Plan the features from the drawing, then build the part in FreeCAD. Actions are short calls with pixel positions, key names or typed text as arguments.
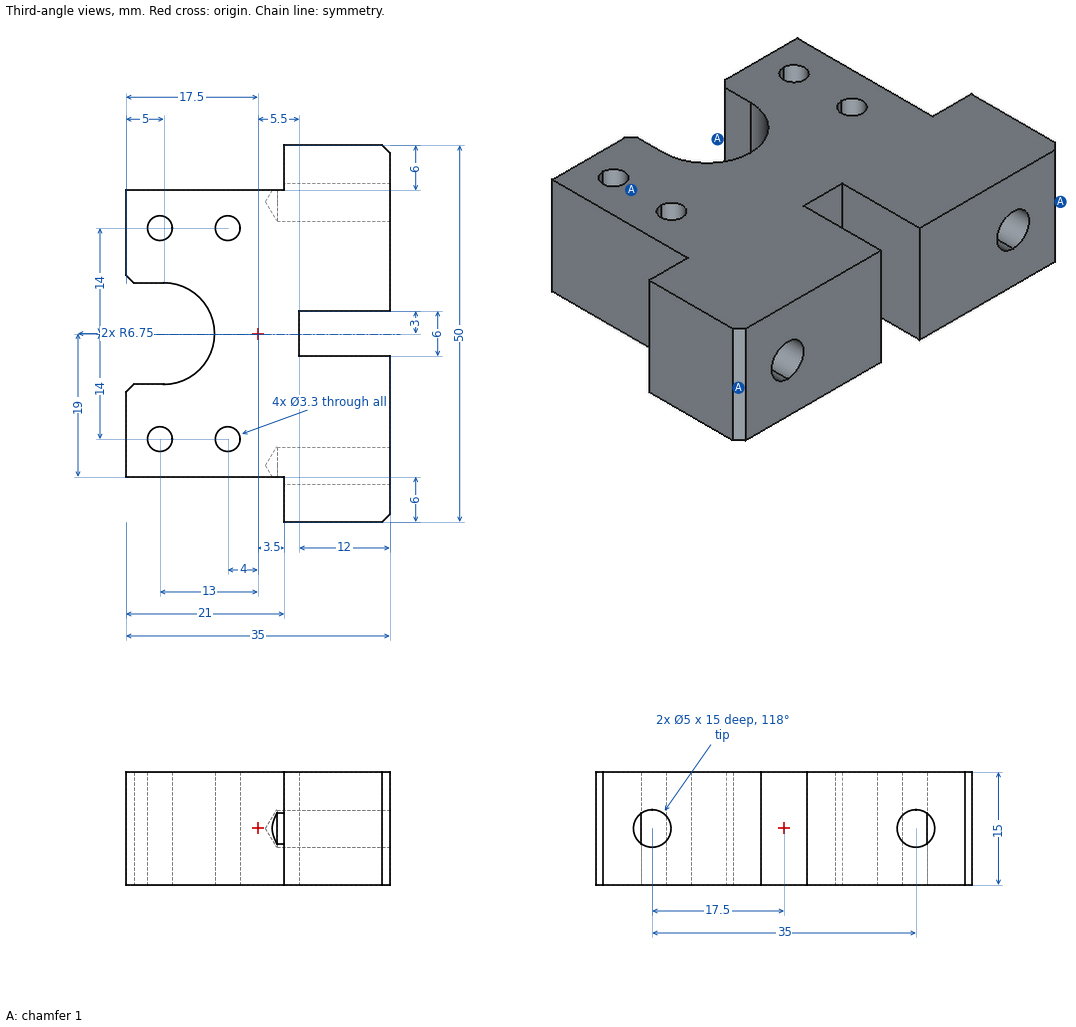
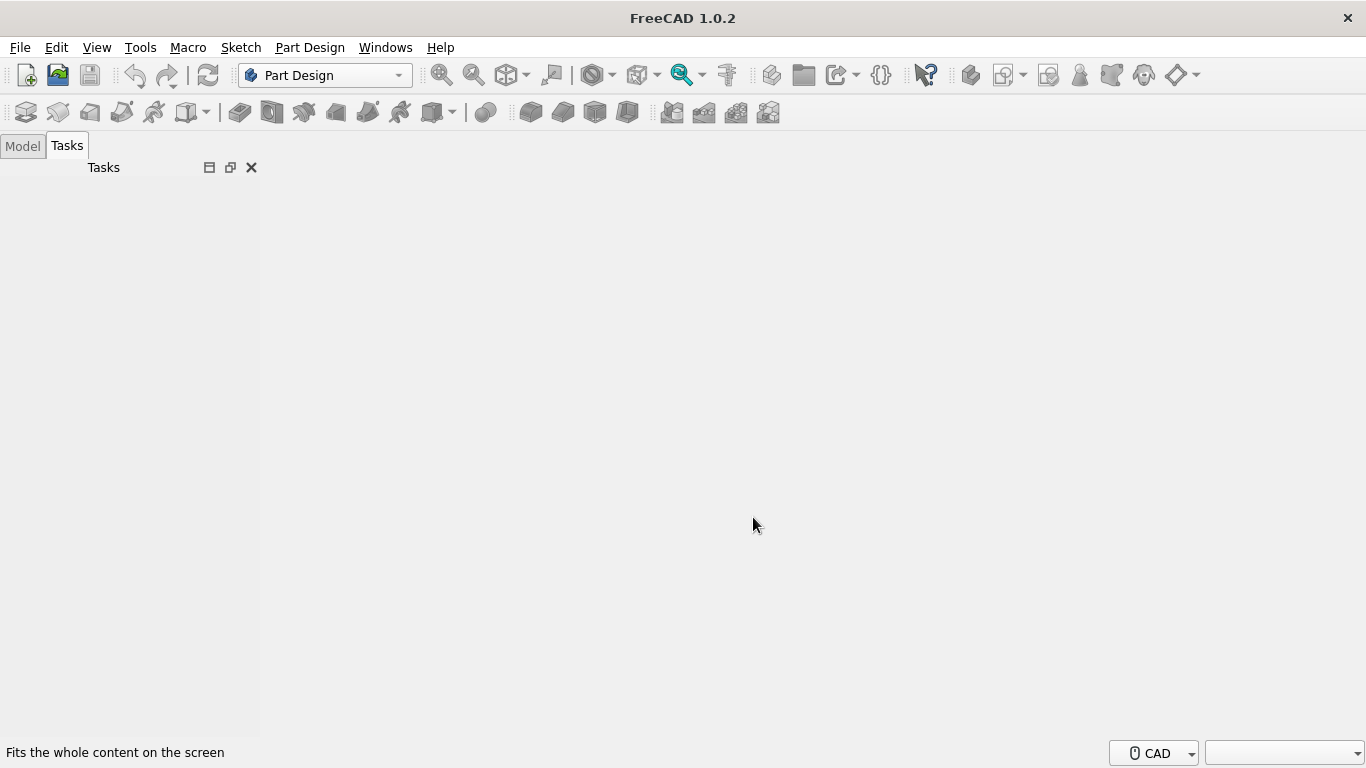
click(26, 76)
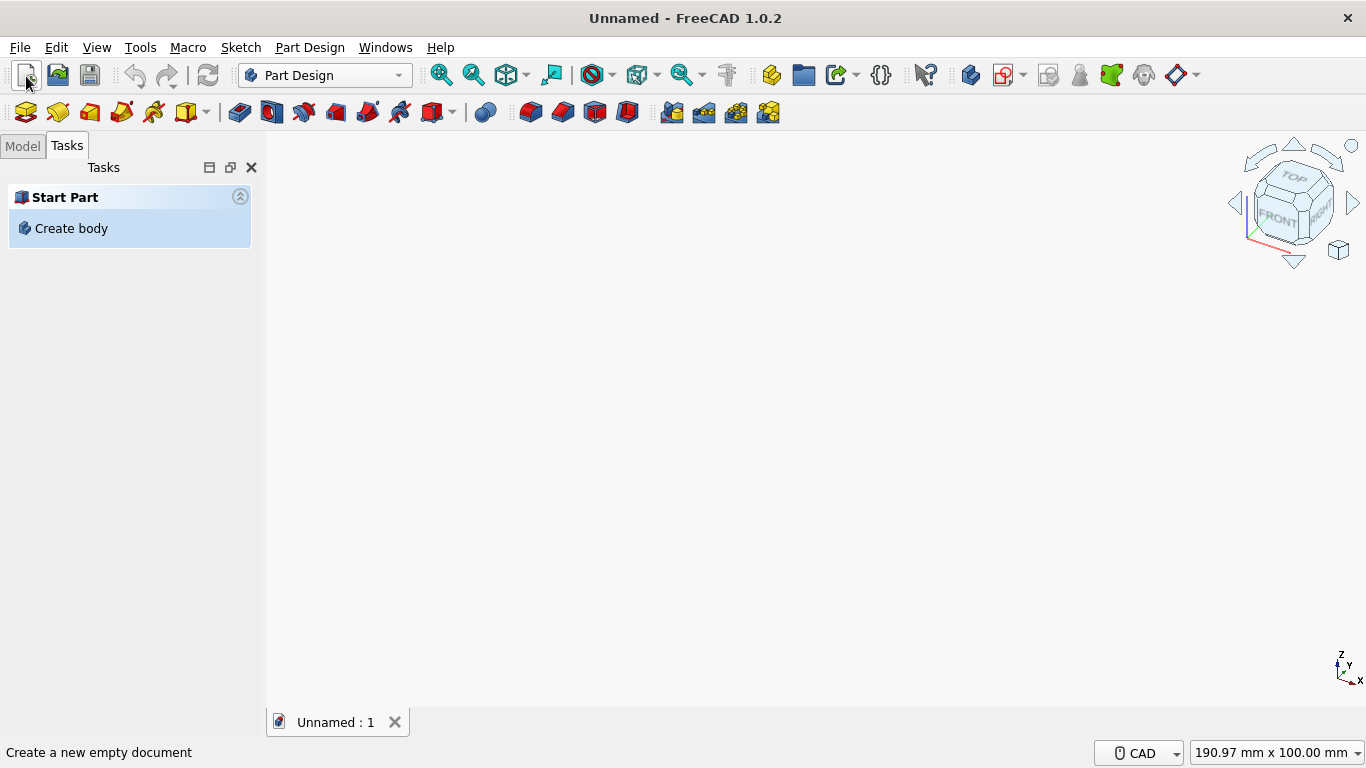
click(1004, 76)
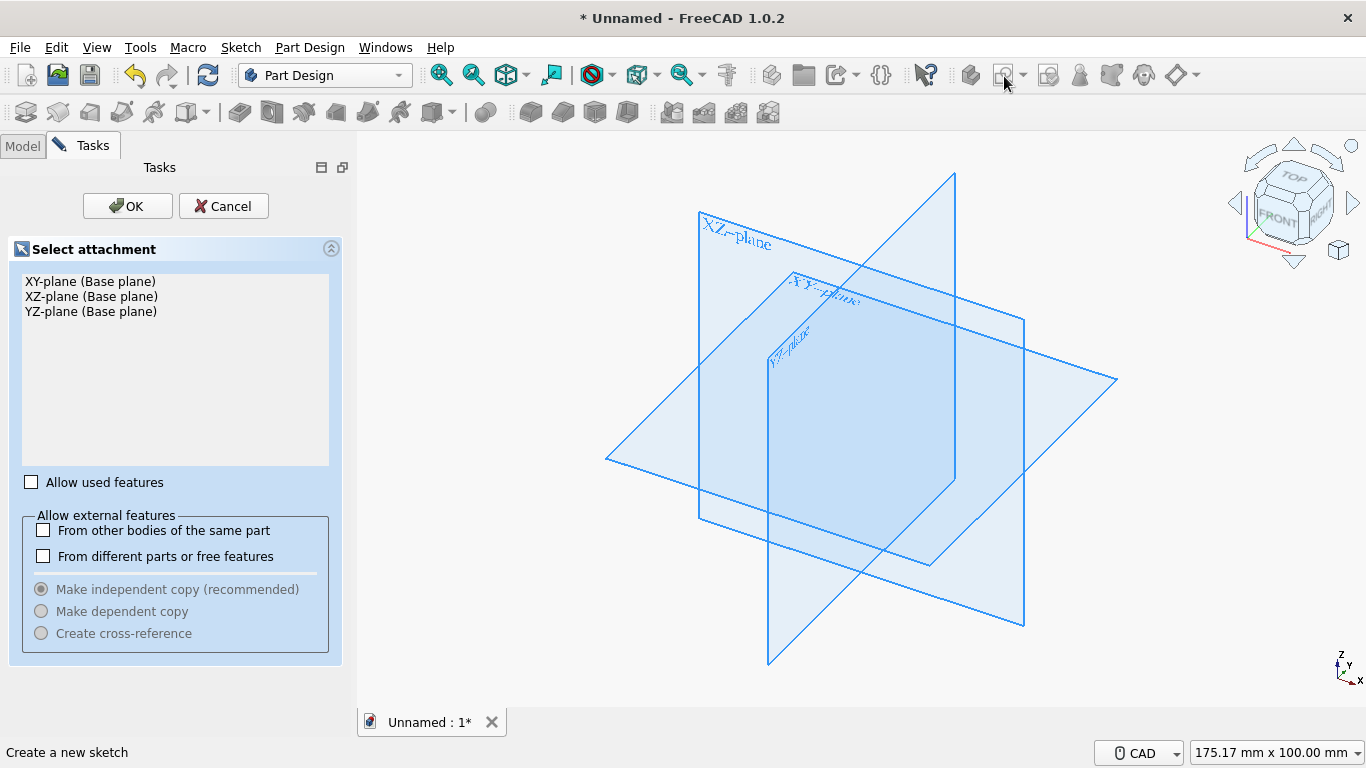
click(82, 282)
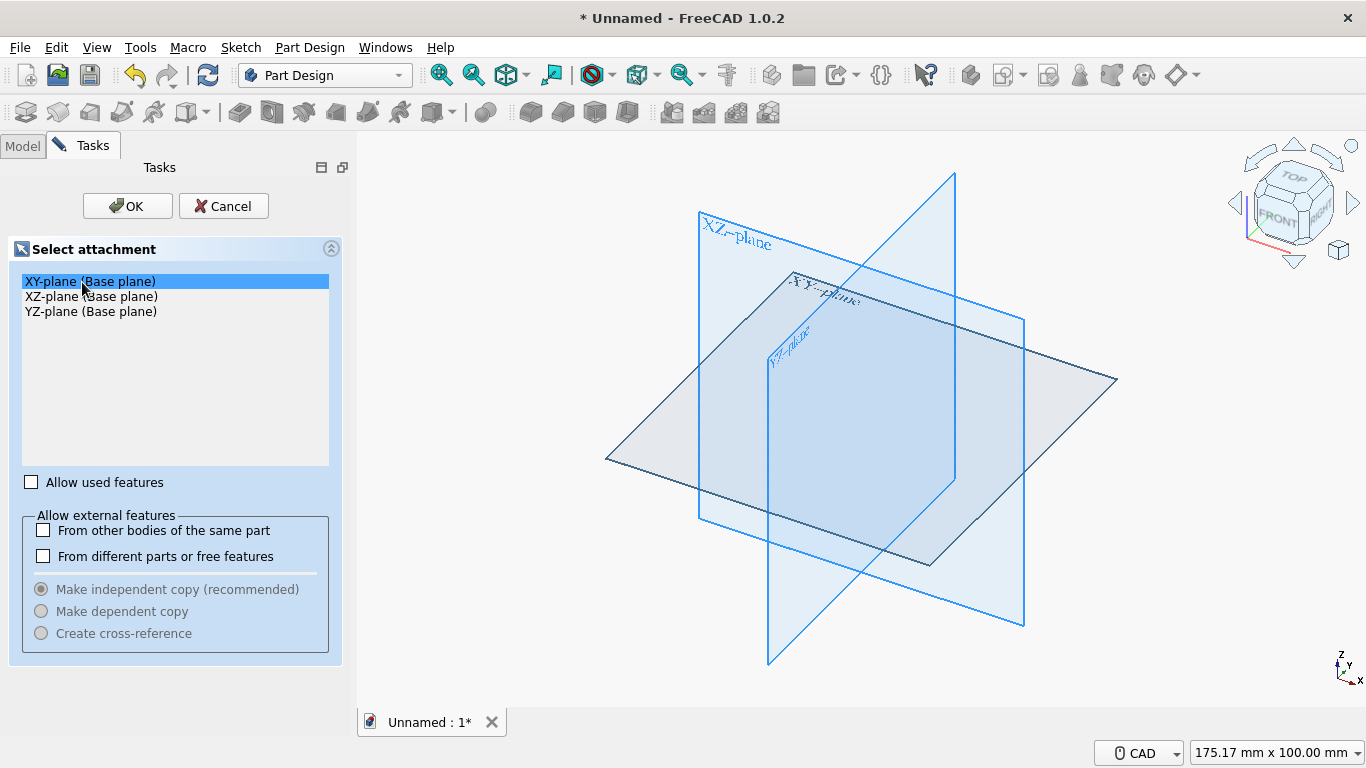
click(128, 206)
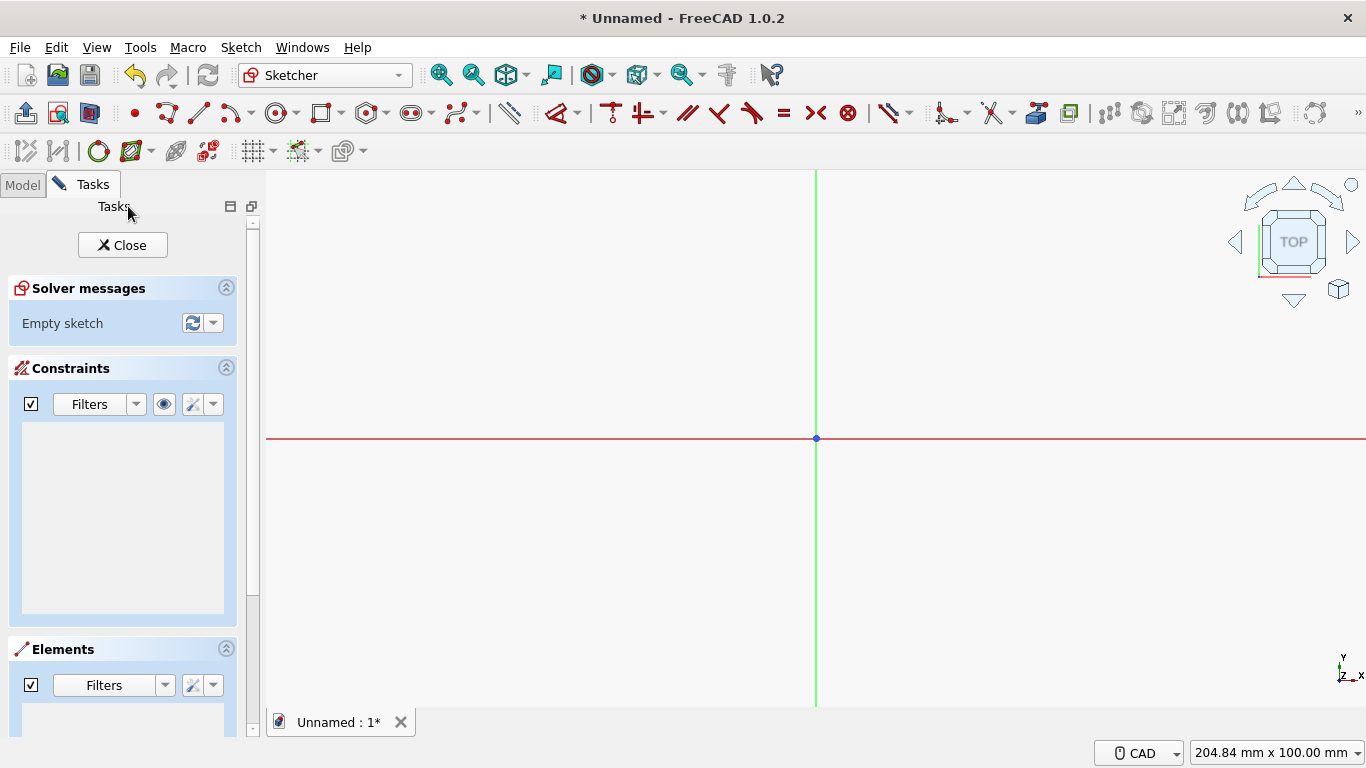
click(344, 114)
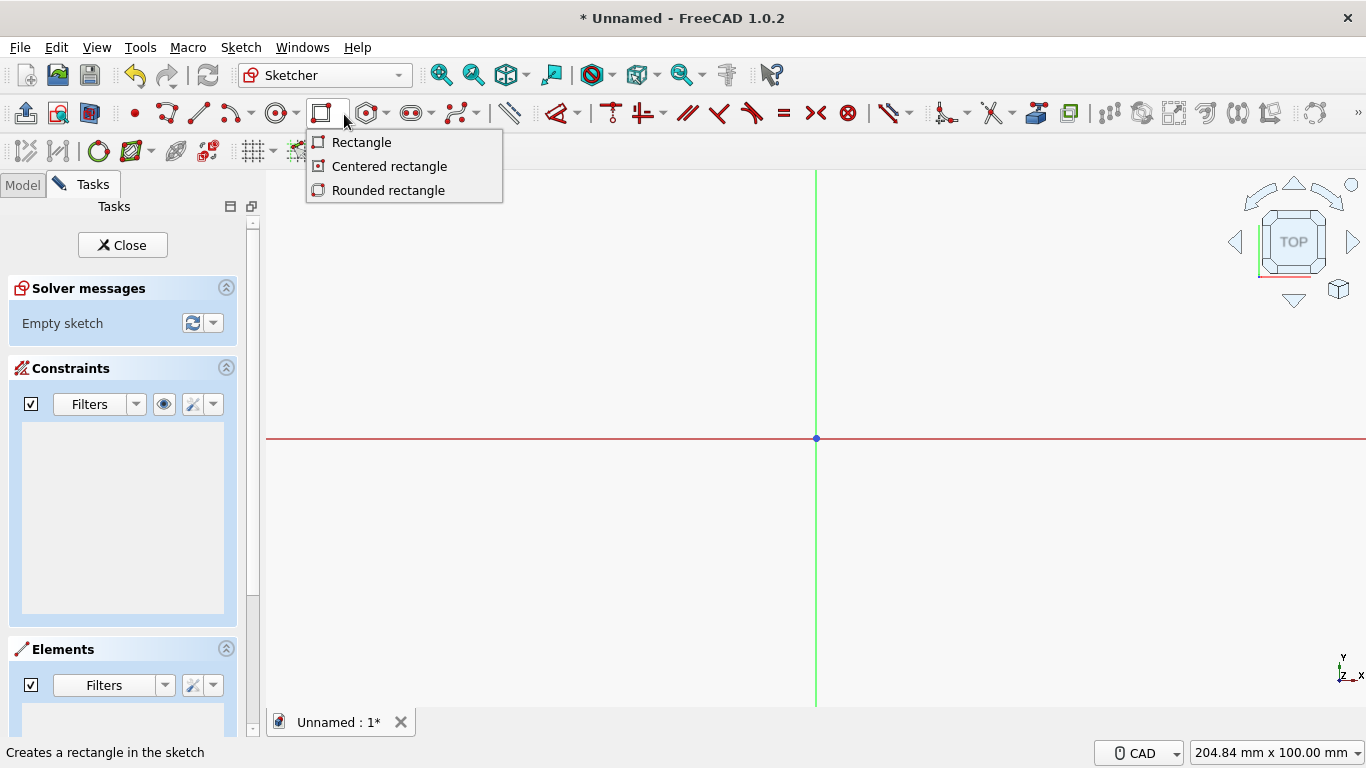
click(404, 166)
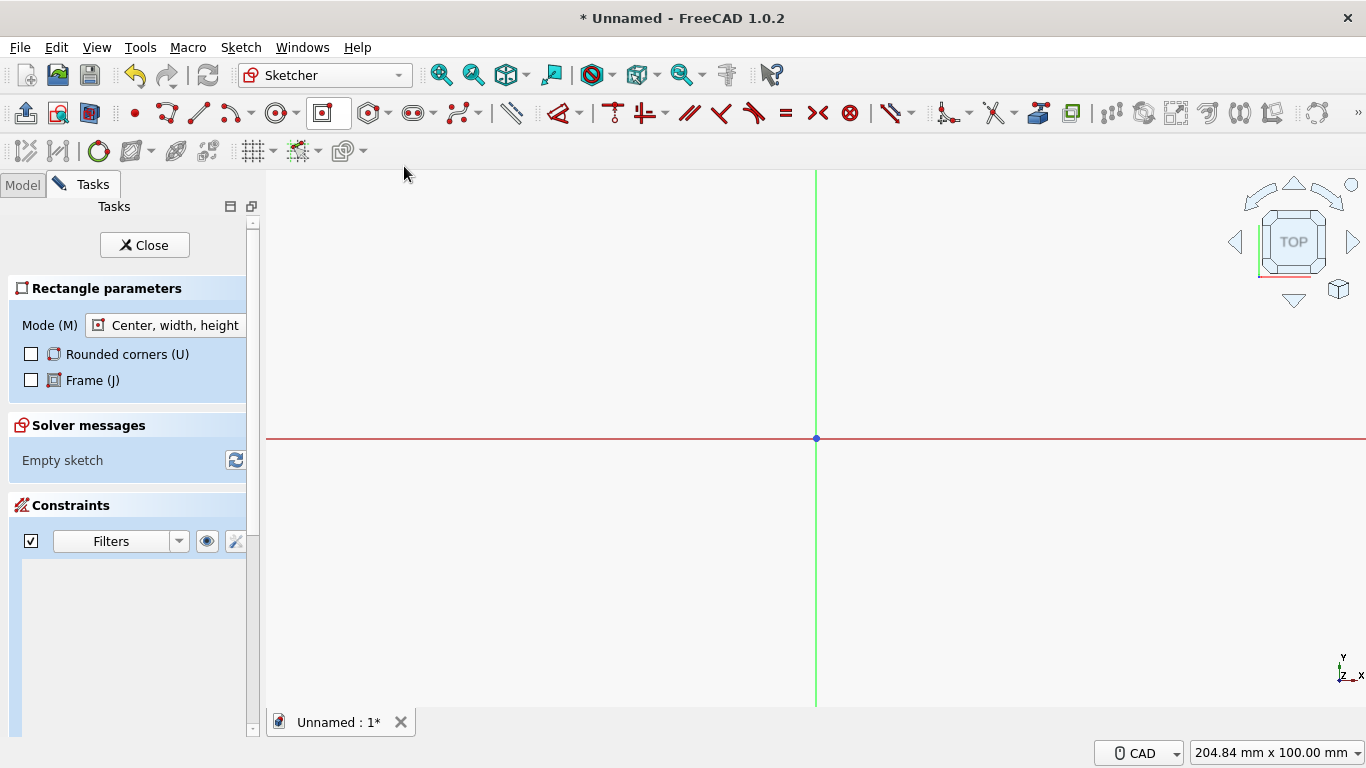
click(816, 438)
move(910, 304)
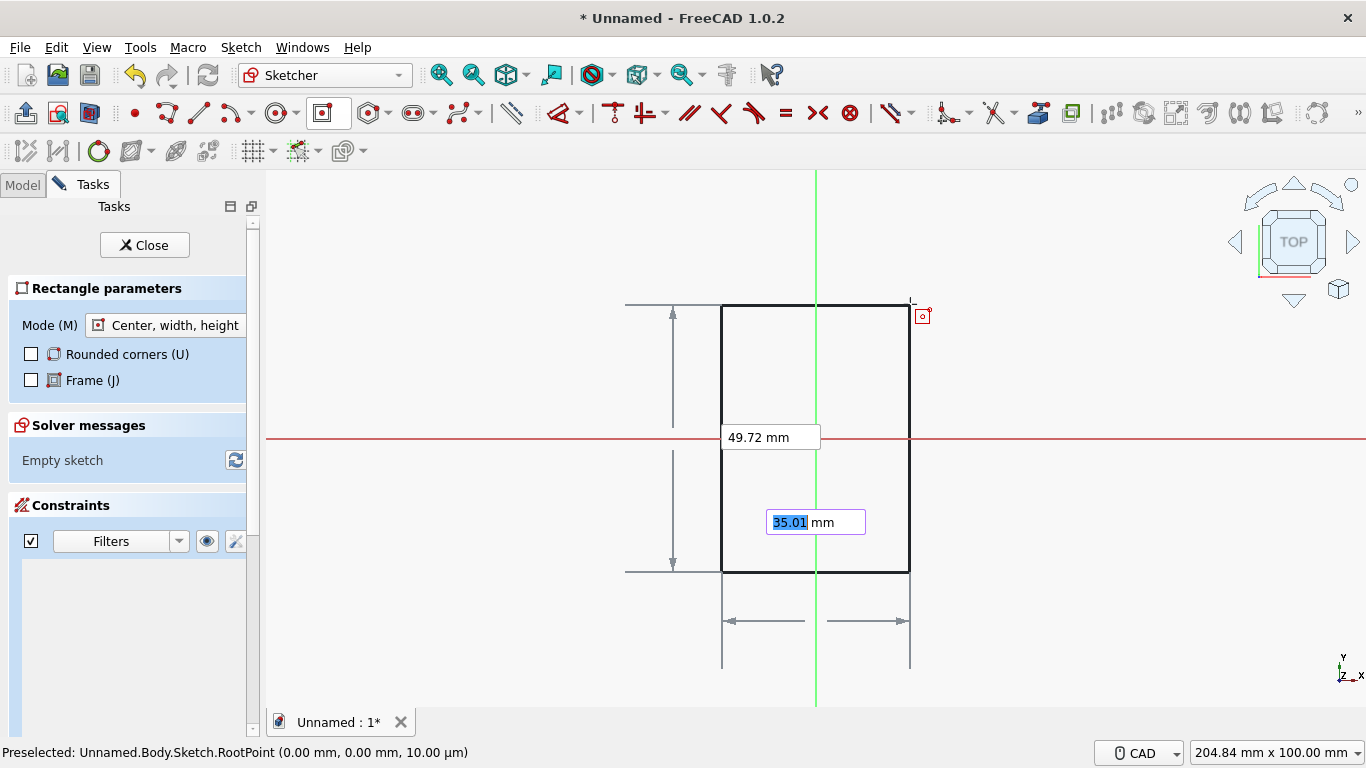
text(35)
key(Tab)
text(50)
key(Return)
key(Escape)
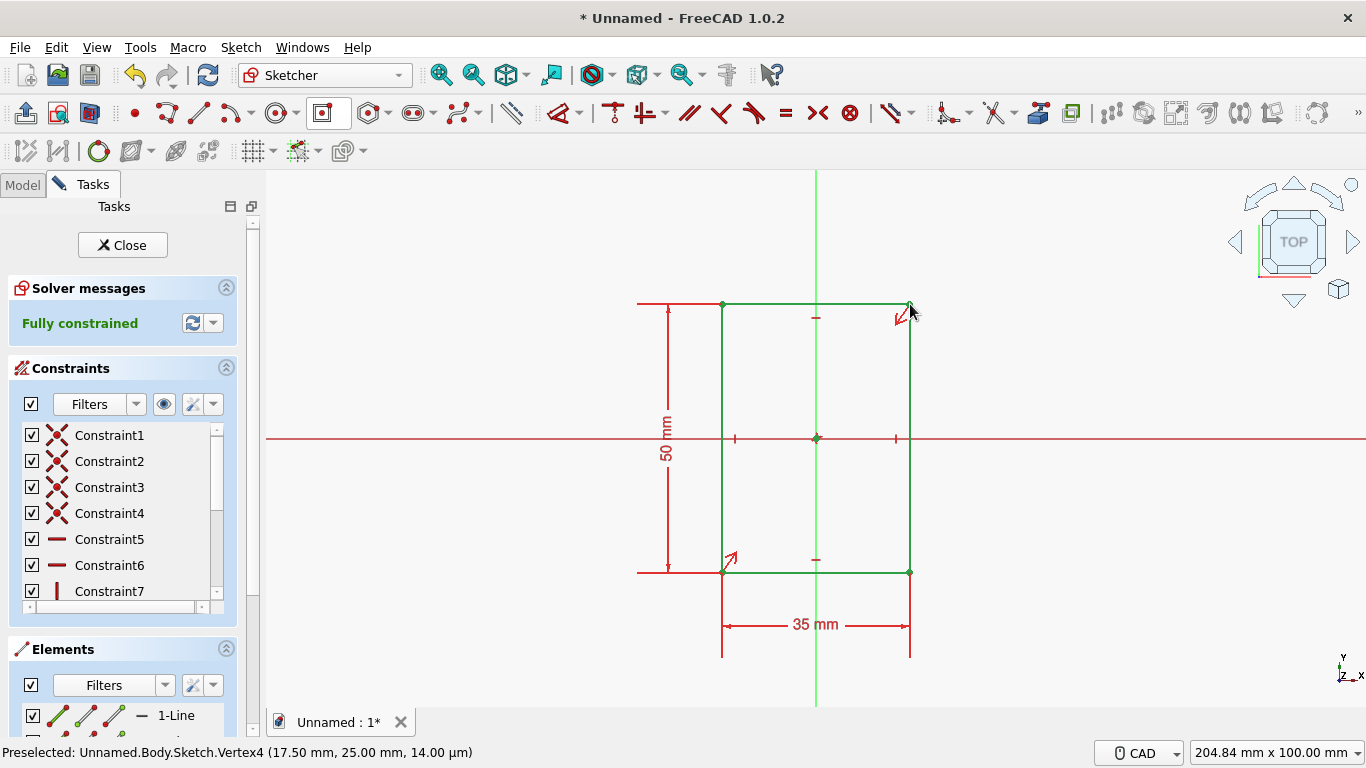
click(123, 245)